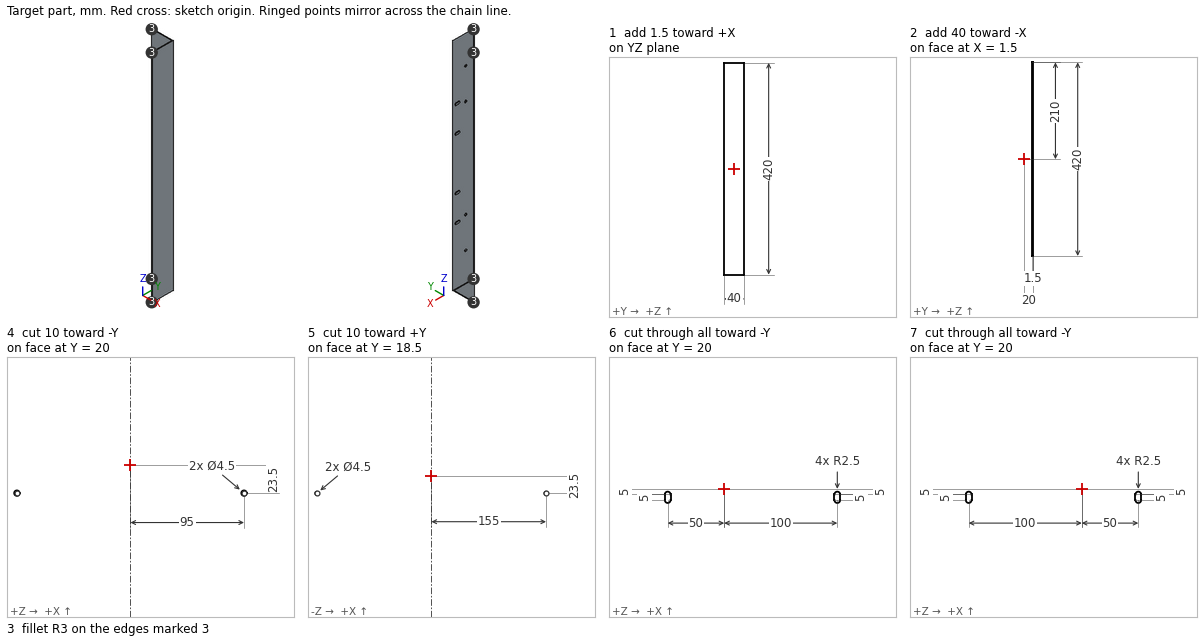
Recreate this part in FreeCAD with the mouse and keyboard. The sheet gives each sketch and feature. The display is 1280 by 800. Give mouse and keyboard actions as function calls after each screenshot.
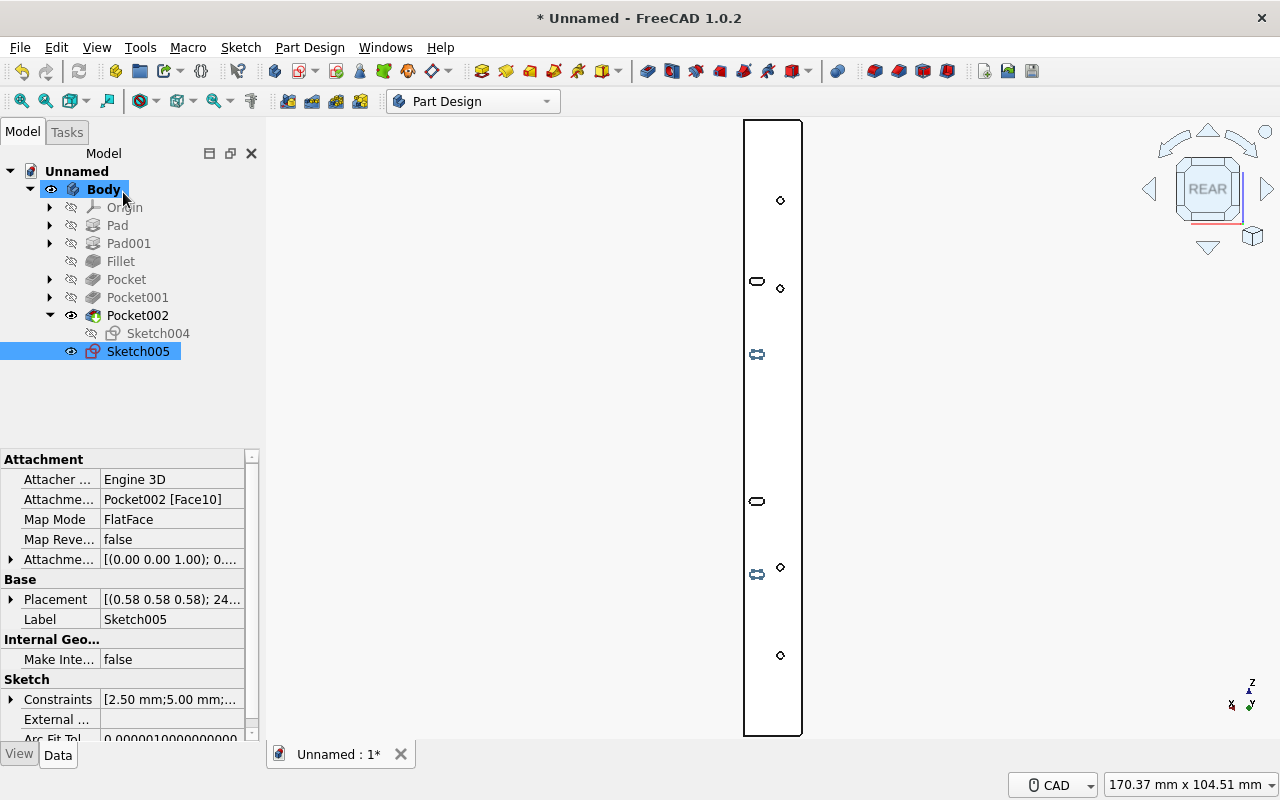
click(648, 72)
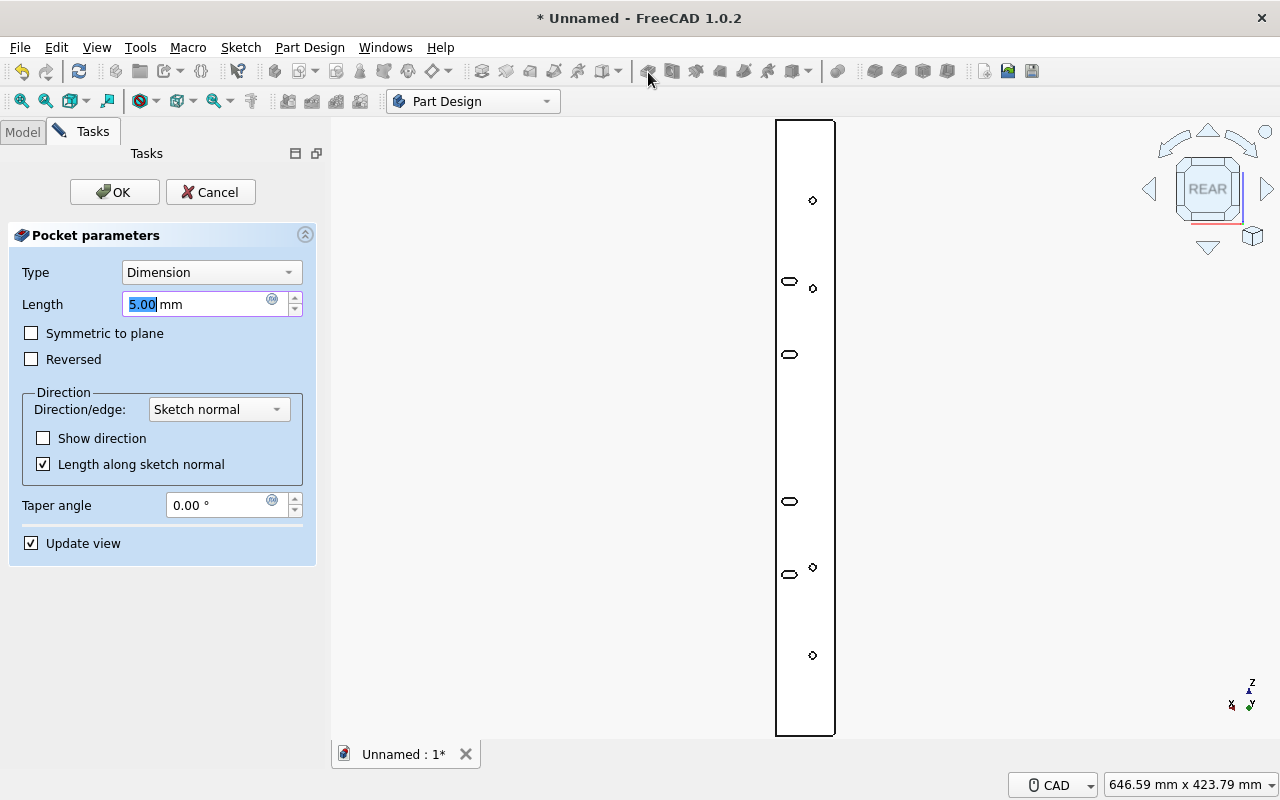
click(212, 272)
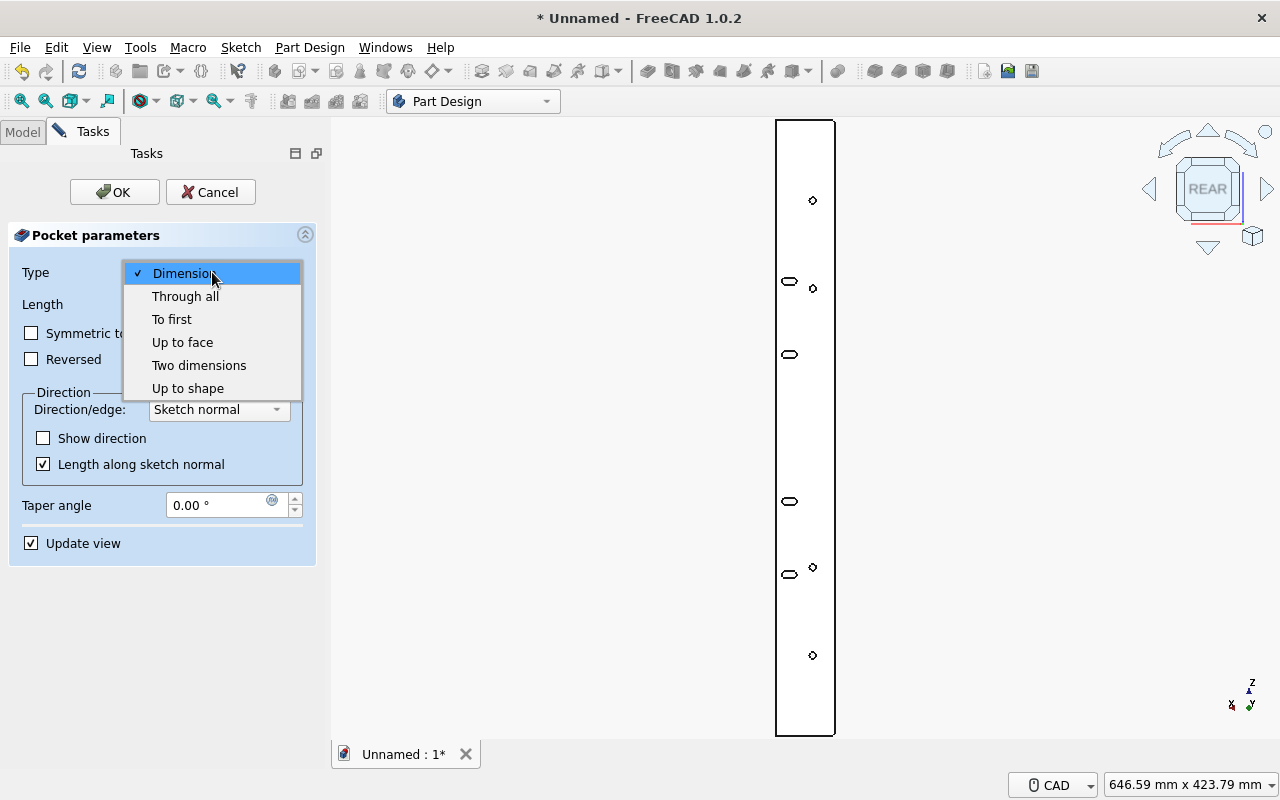
click(212, 296)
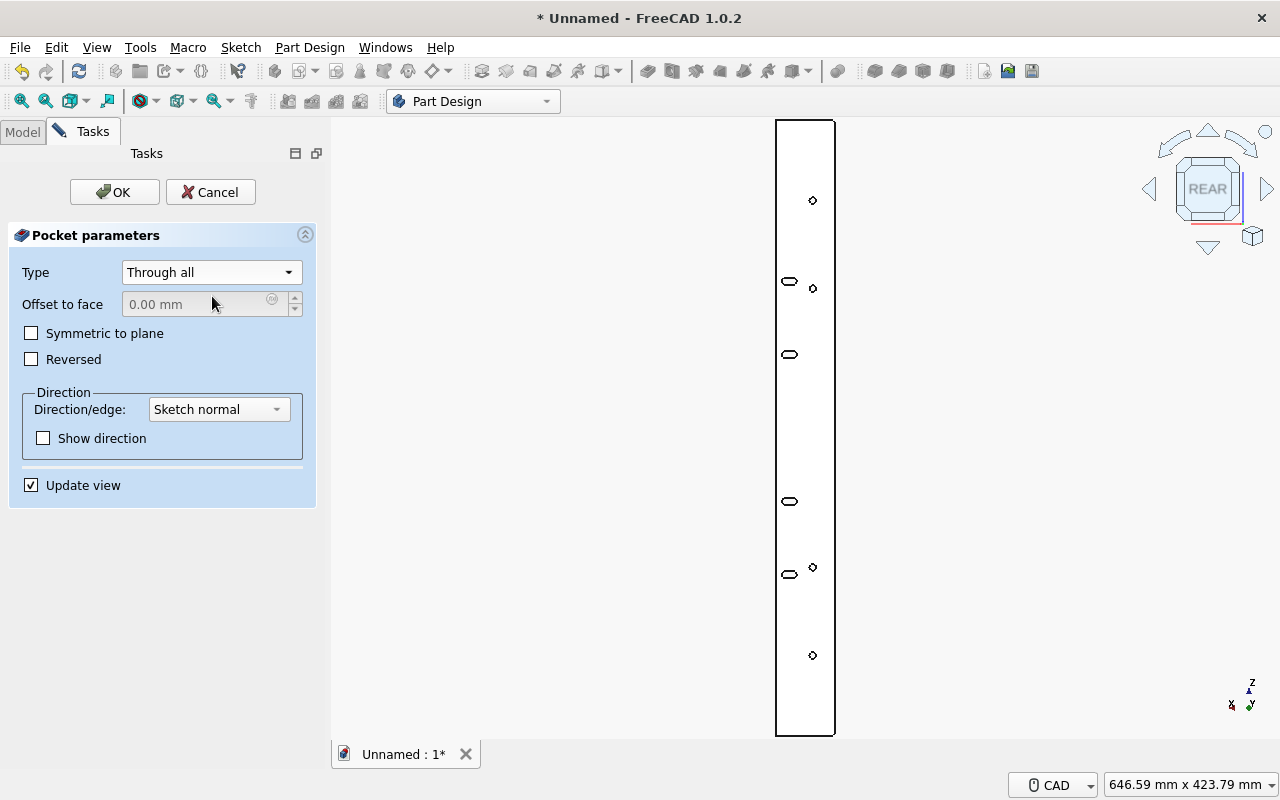
click(115, 192)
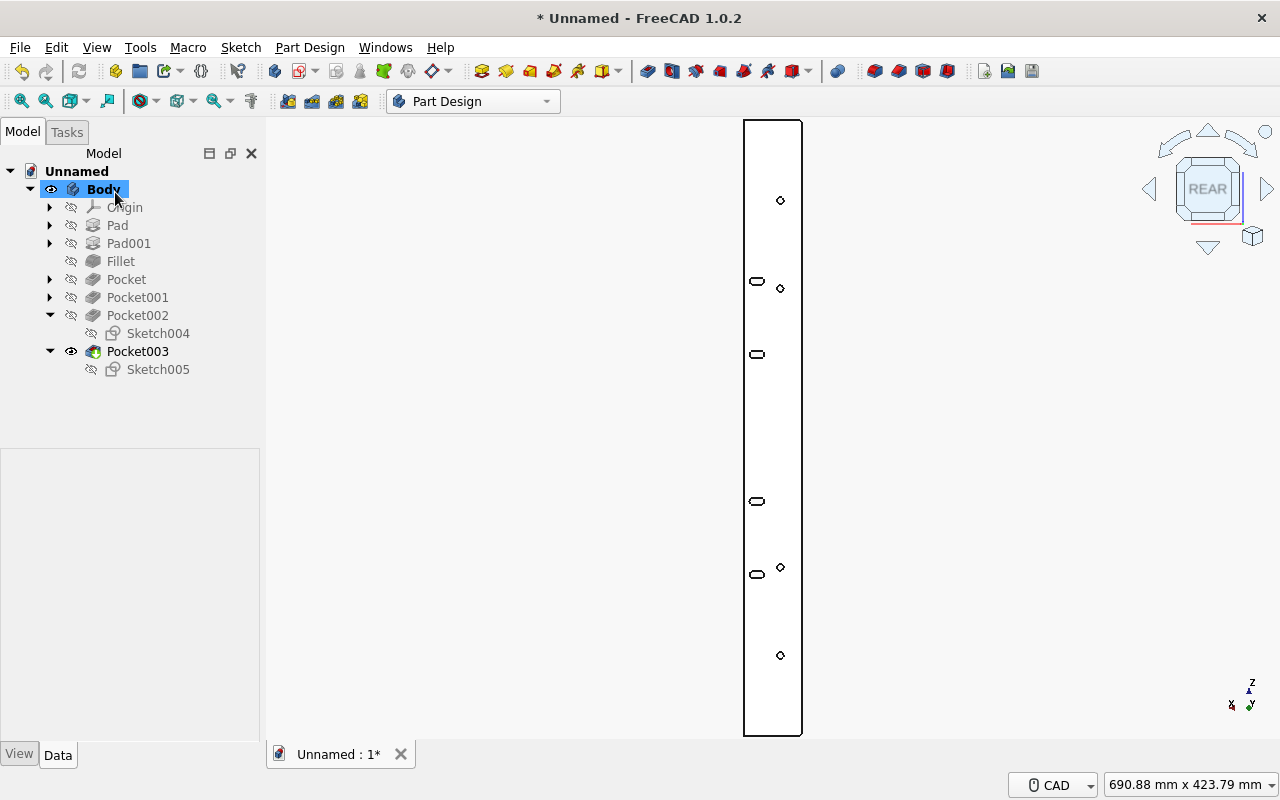
key(0)